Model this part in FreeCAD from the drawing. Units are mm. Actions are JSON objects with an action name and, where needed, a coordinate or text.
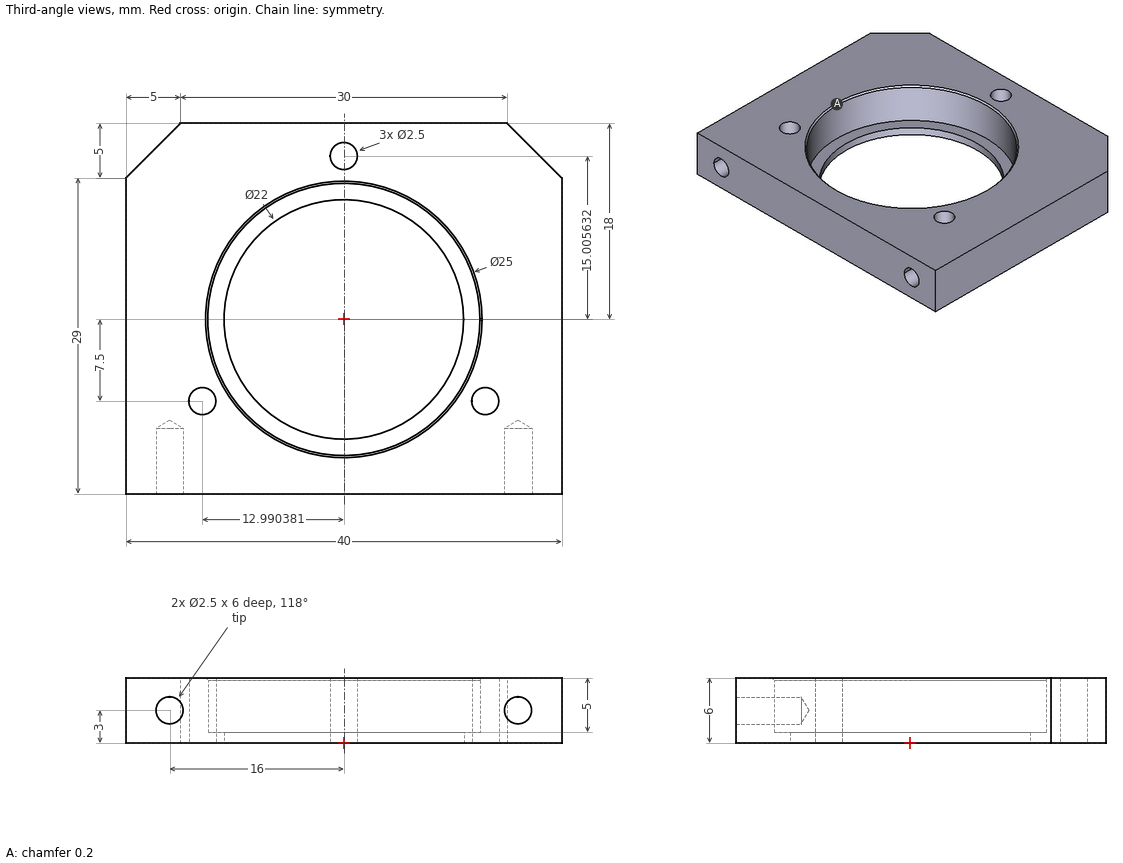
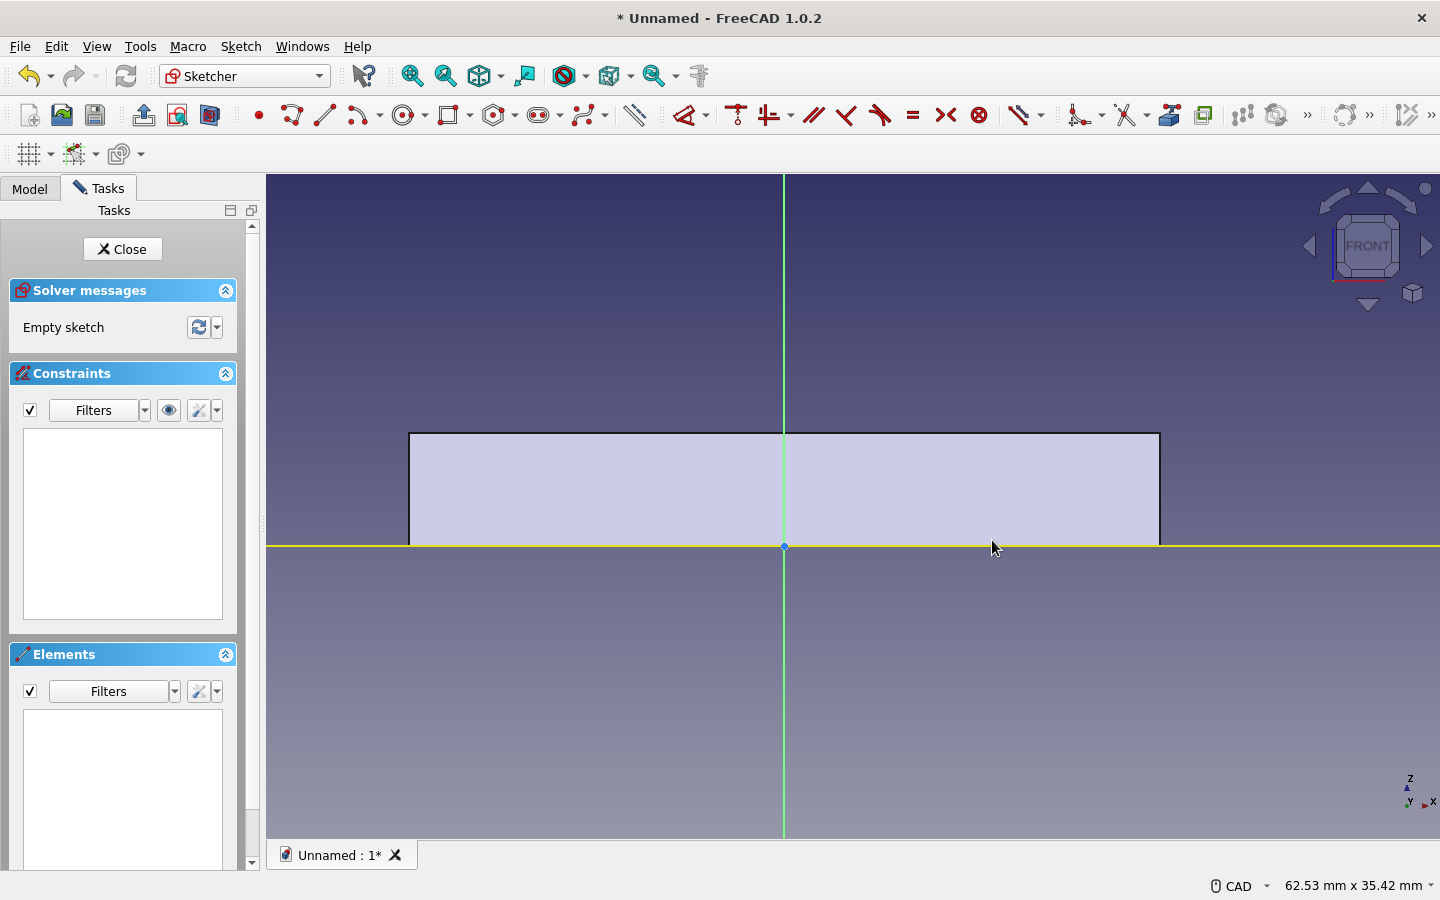
{"action": "left_click", "coordinate": [402, 116]}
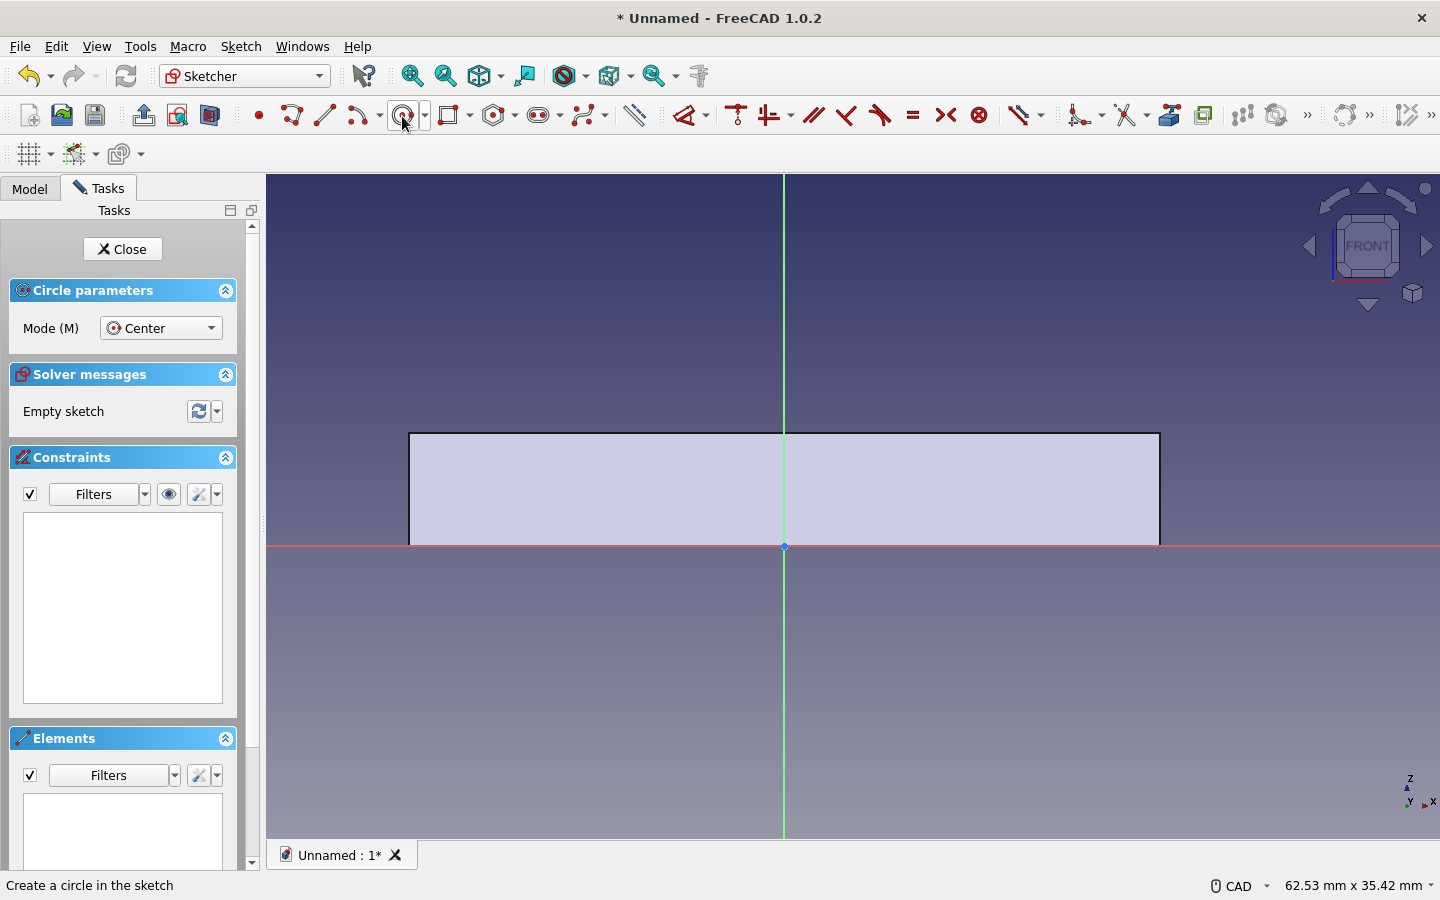
{"action": "left_click", "coordinate": [484, 490]}
{"action": "left_click", "coordinate": [501, 473]}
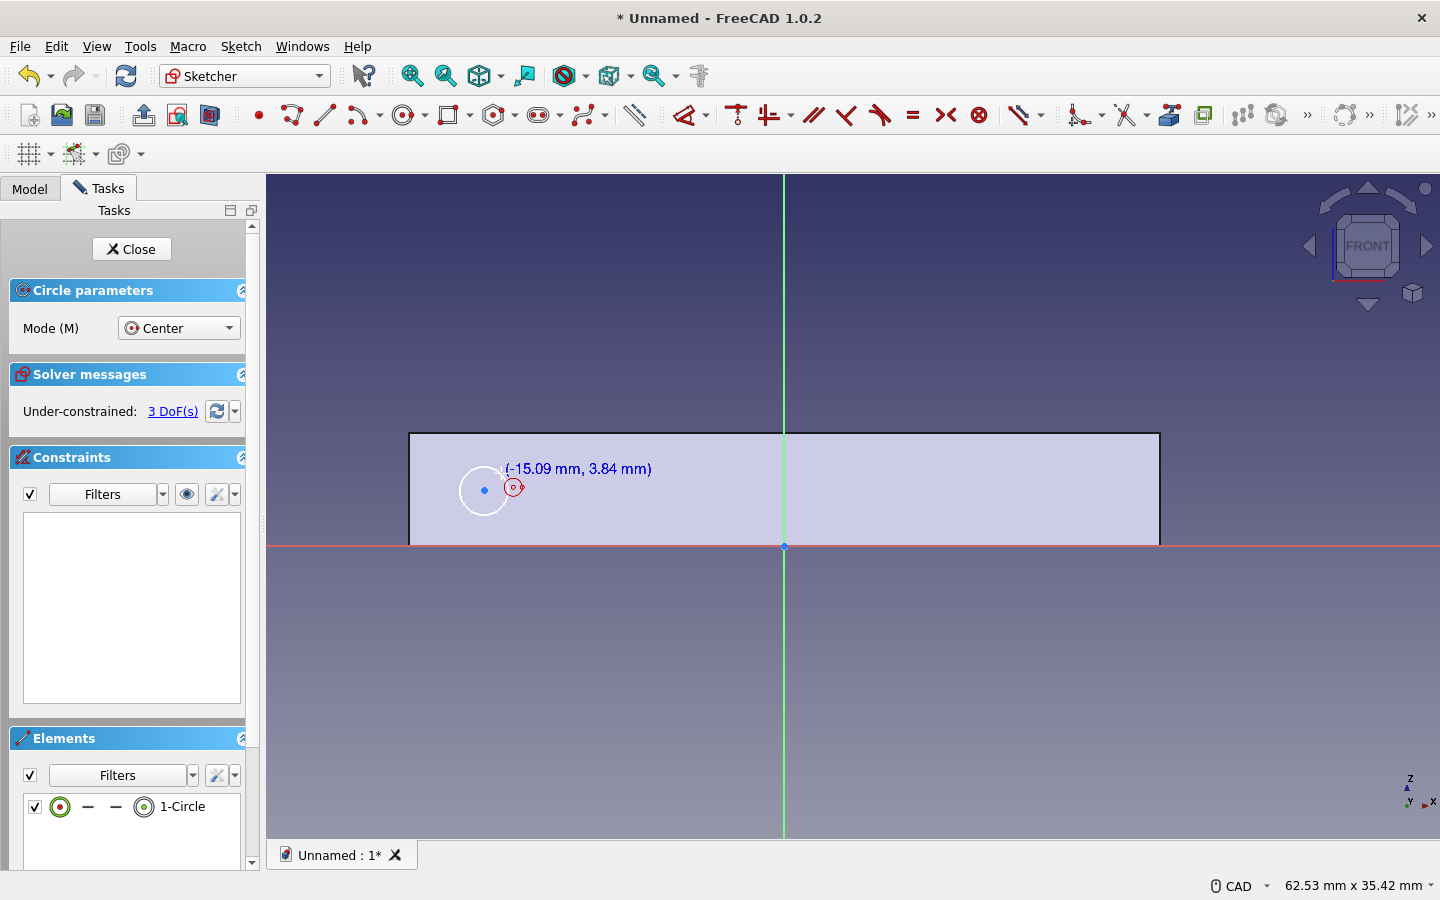
{"action": "left_click", "coordinate": [1085, 490]}
{"action": "left_click", "coordinate": [1101, 473]}
{"action": "key", "text": "Escape"}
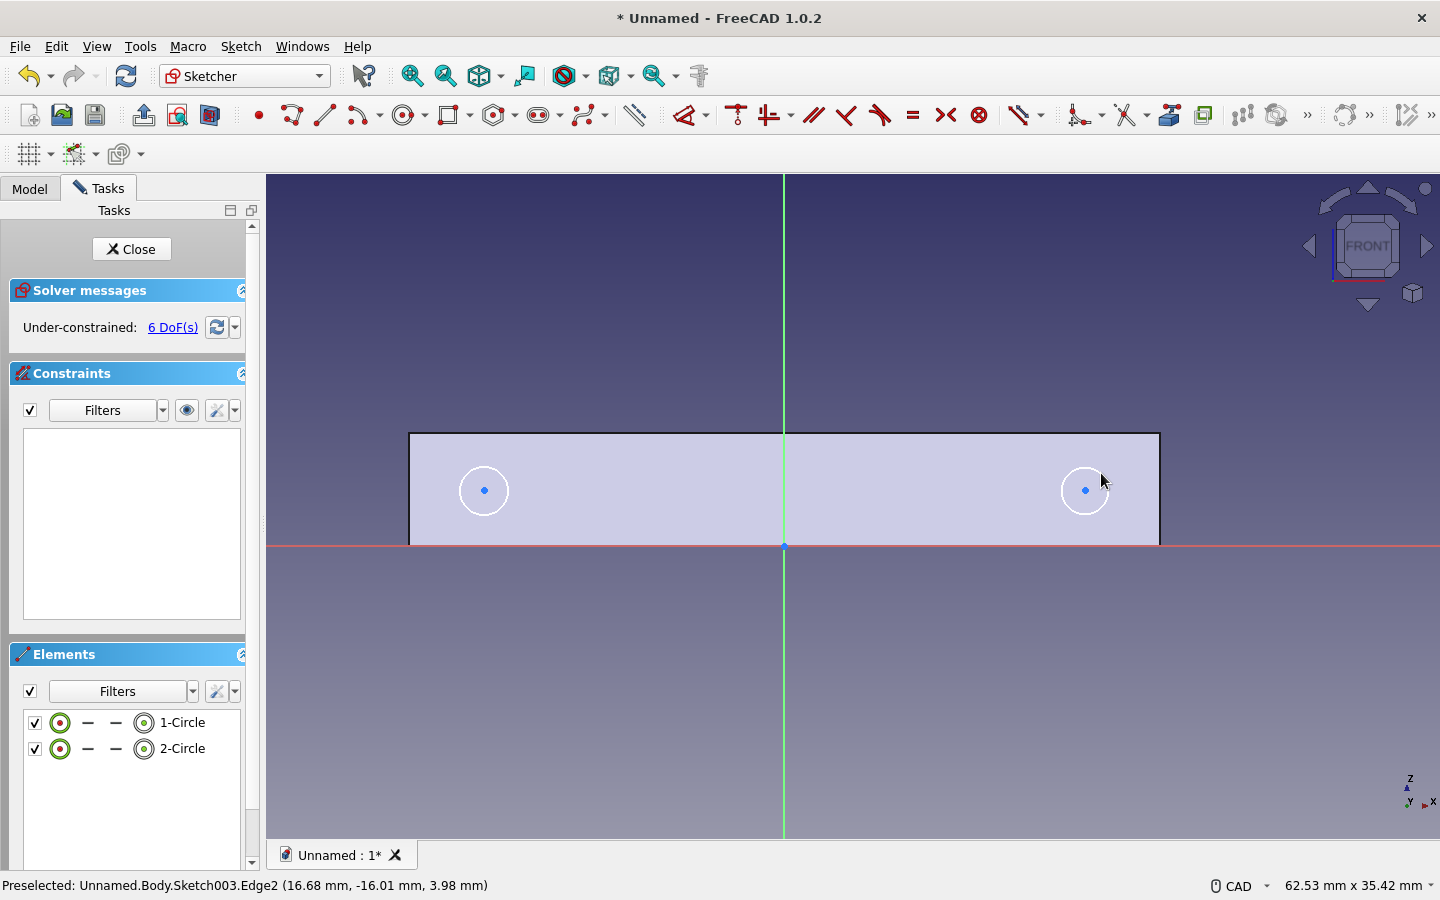
{"action": "left_click", "coordinate": [501, 474]}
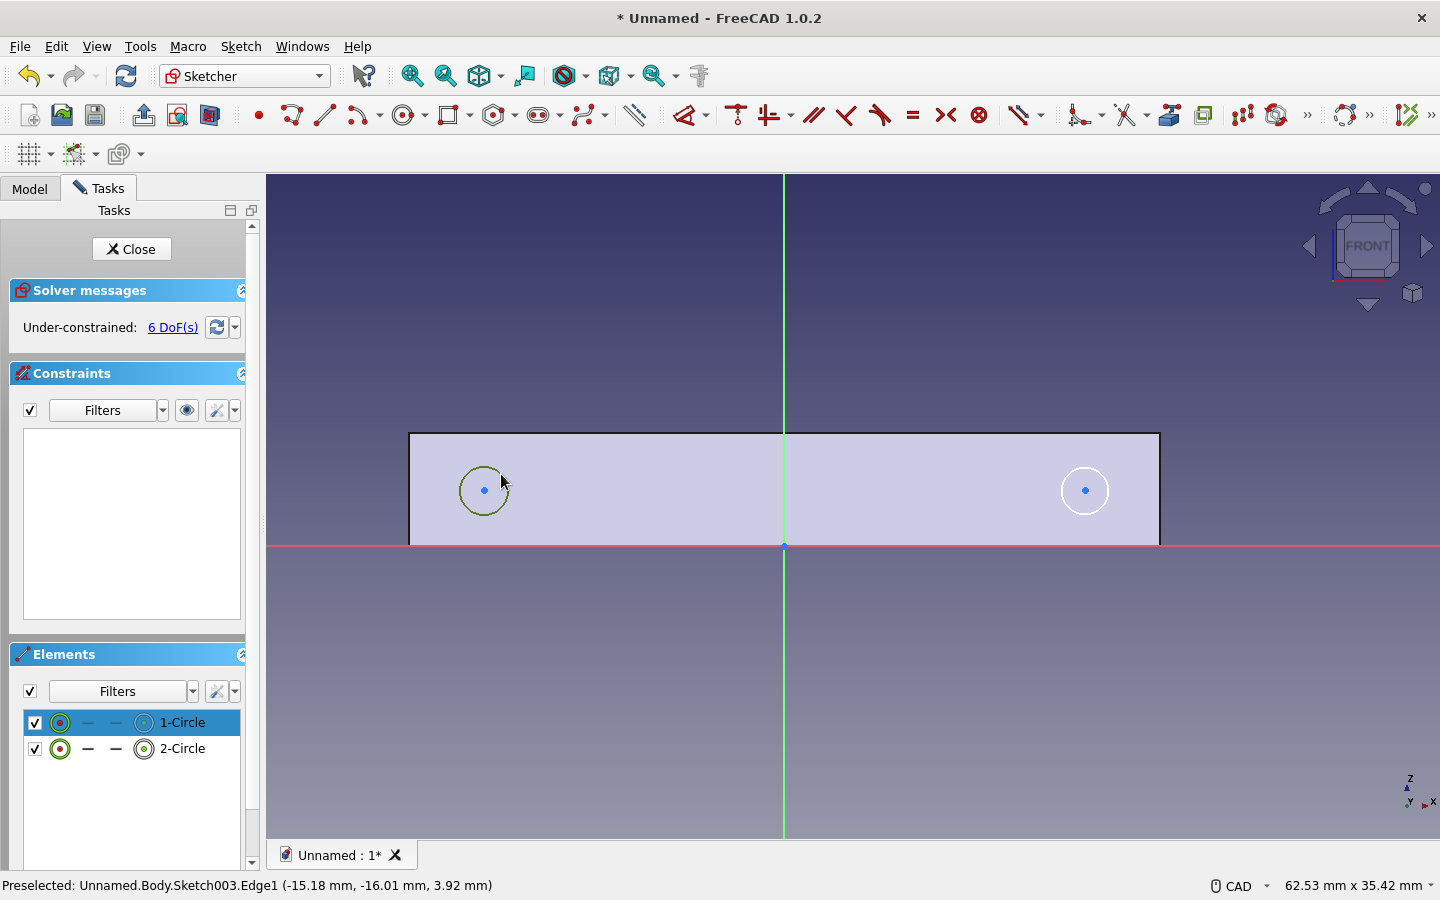
{"action": "left_click", "coordinate": [1101, 474]}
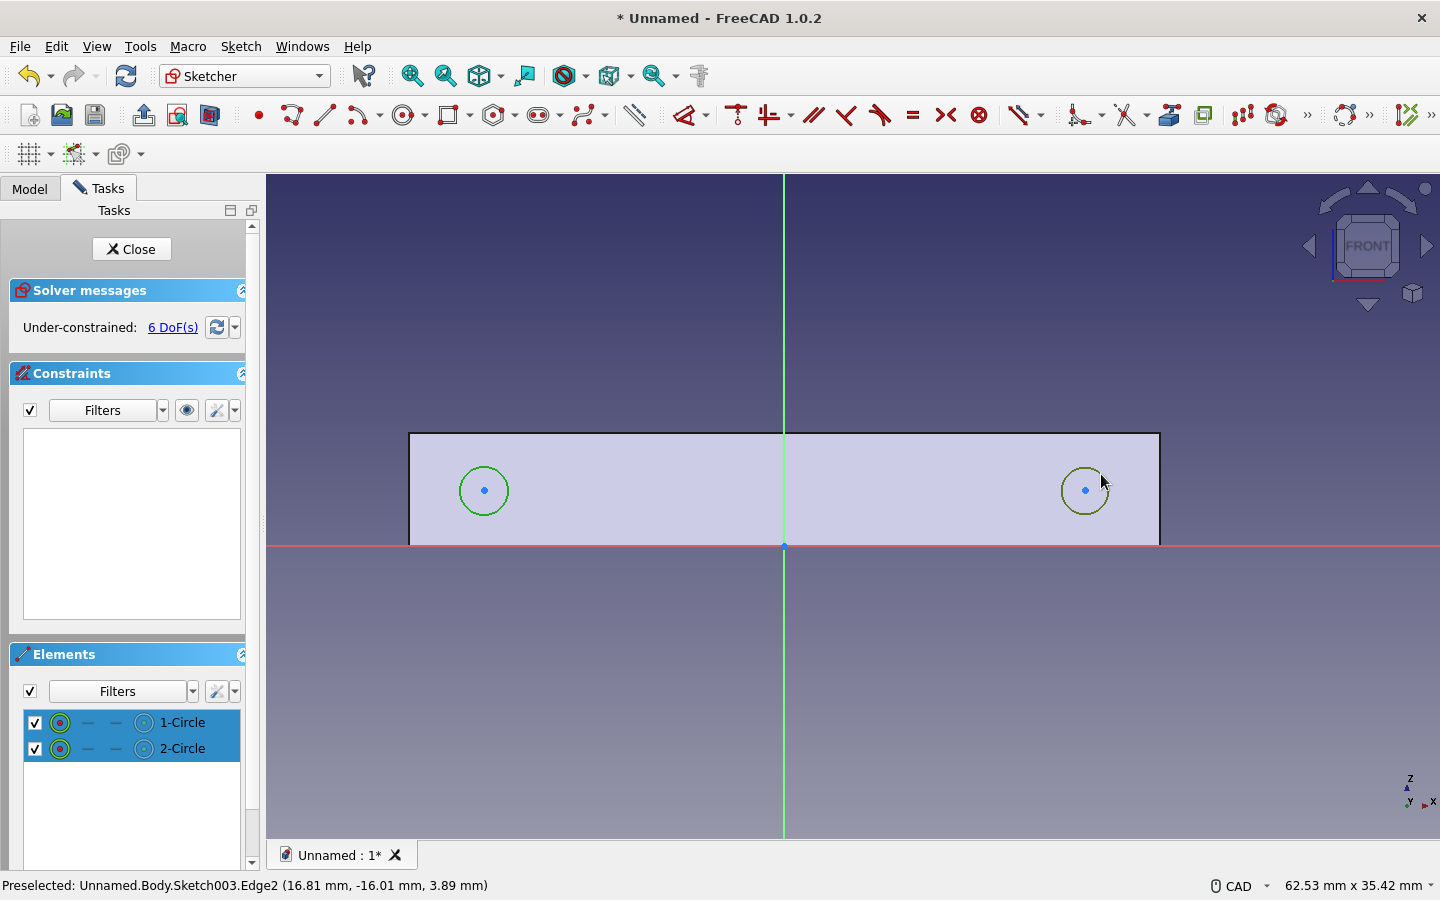
{"action": "key", "text": "e"}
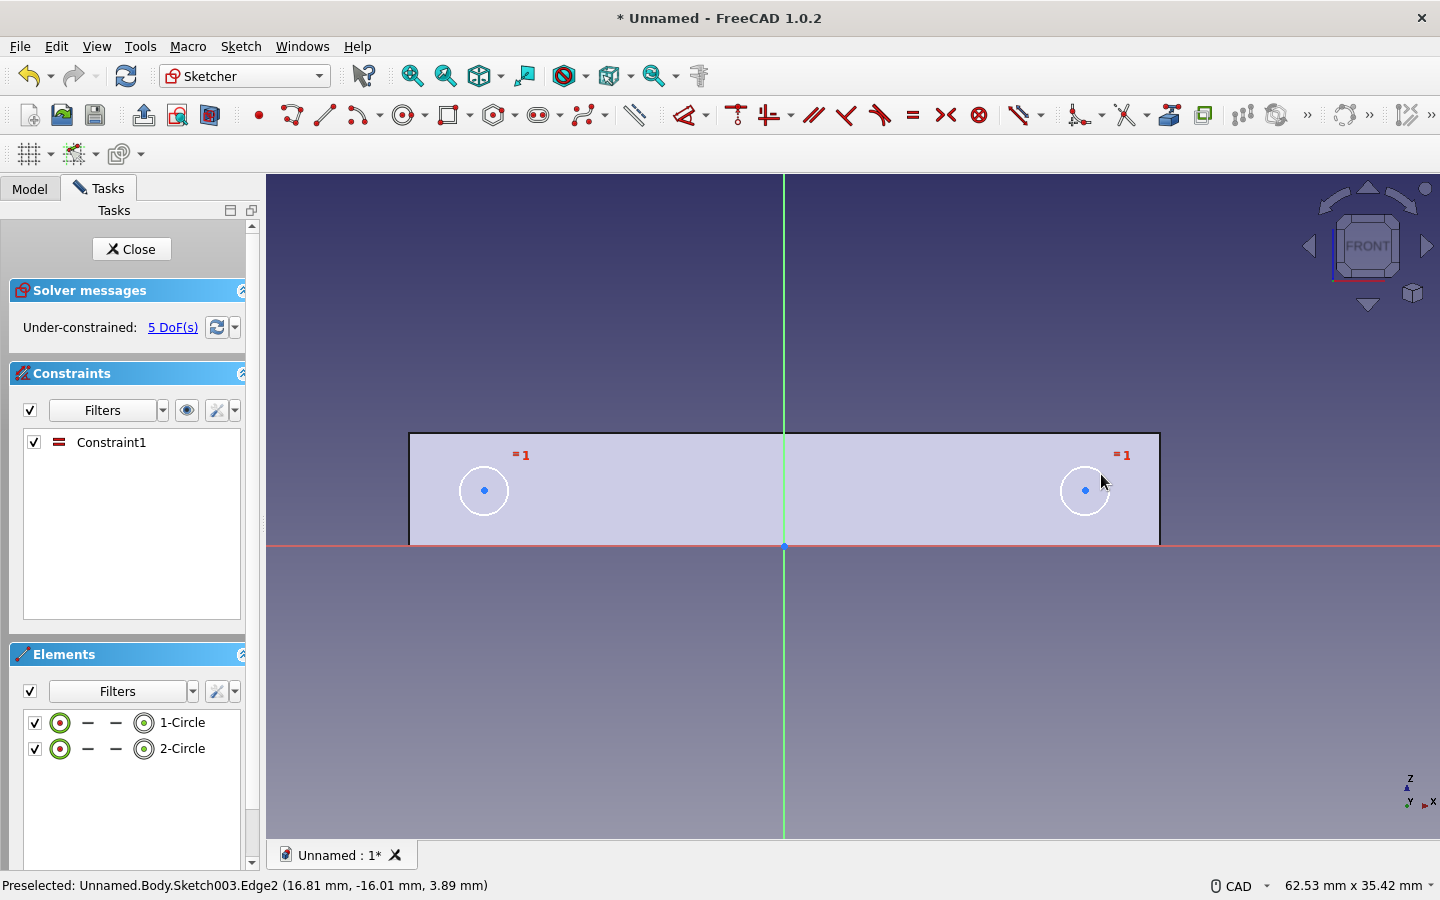
{"action": "left_click", "coordinate": [484, 491]}